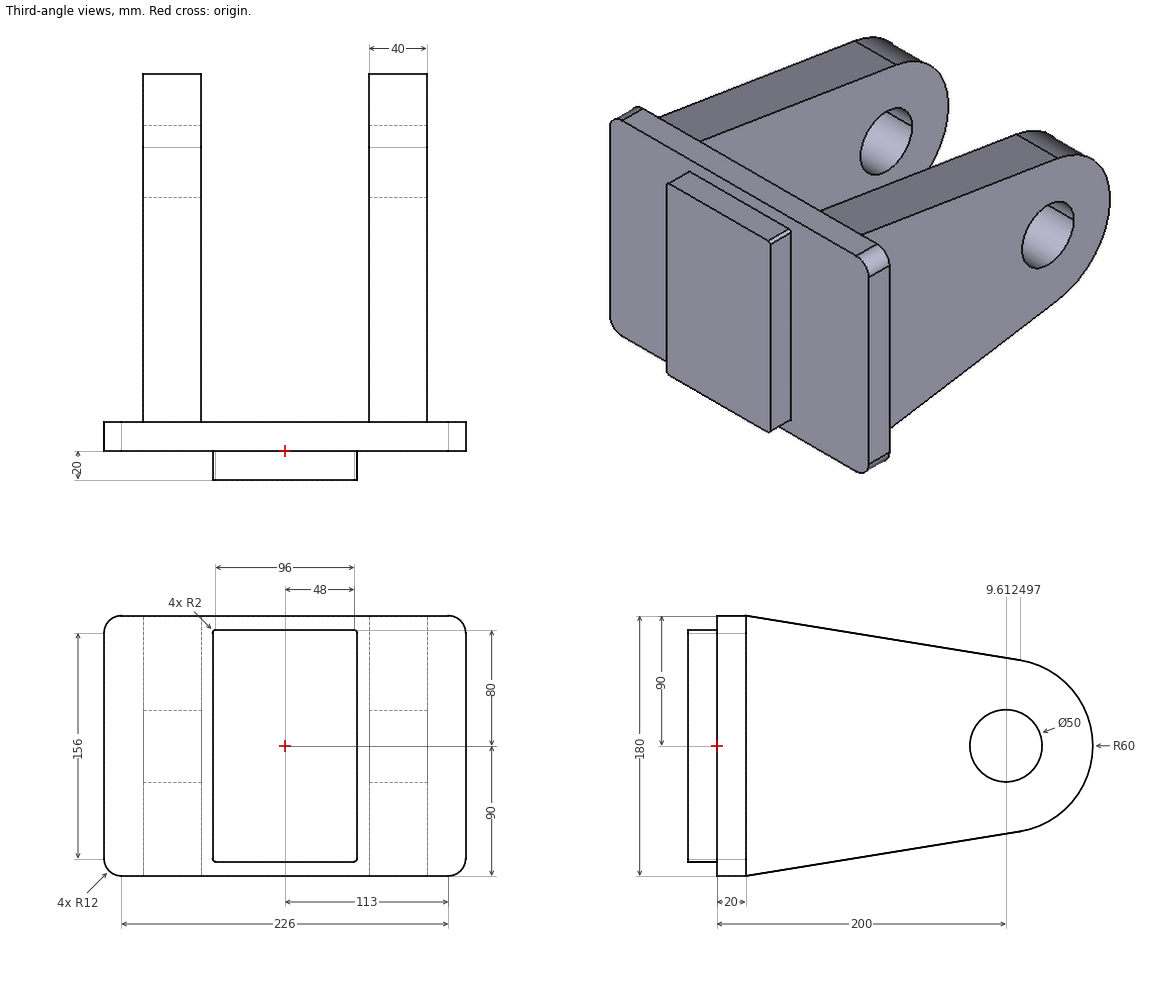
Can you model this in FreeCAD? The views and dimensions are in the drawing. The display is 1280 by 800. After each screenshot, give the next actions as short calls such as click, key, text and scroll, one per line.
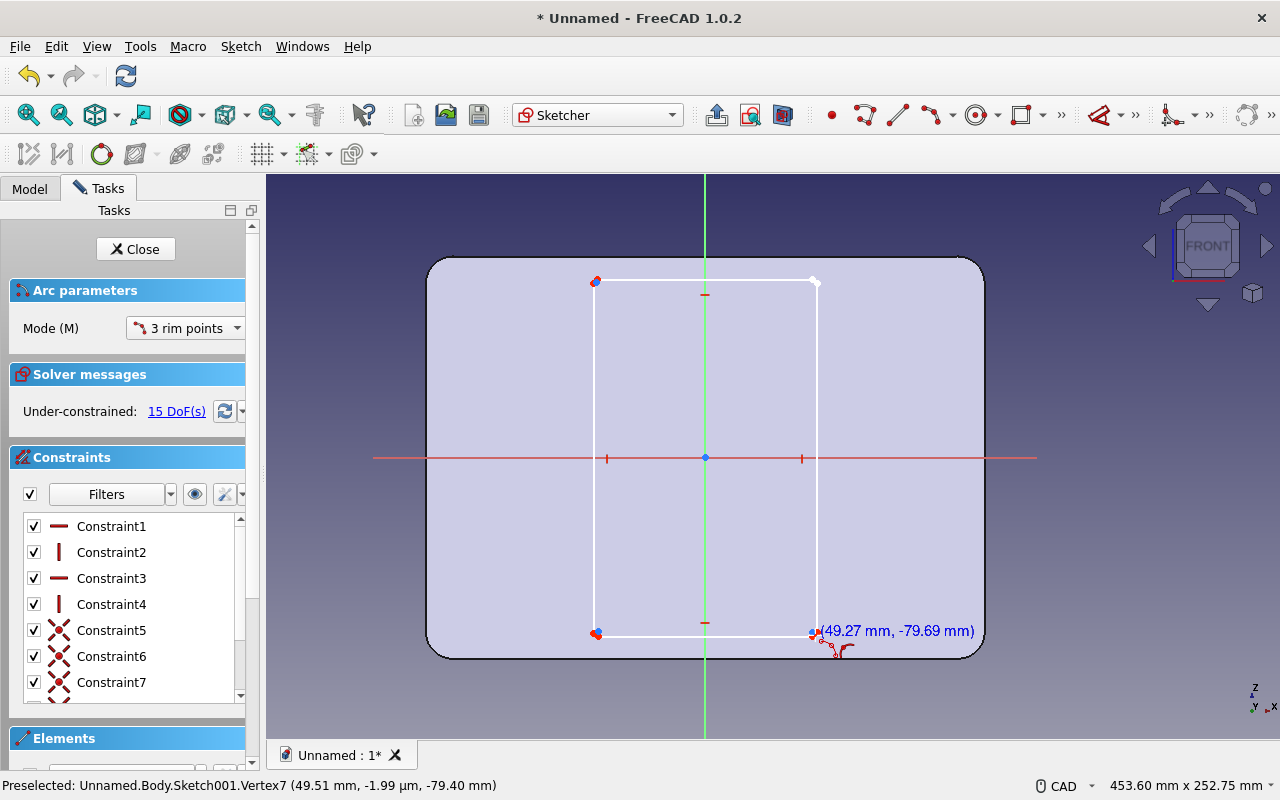
scroll(817, 283, up, 5)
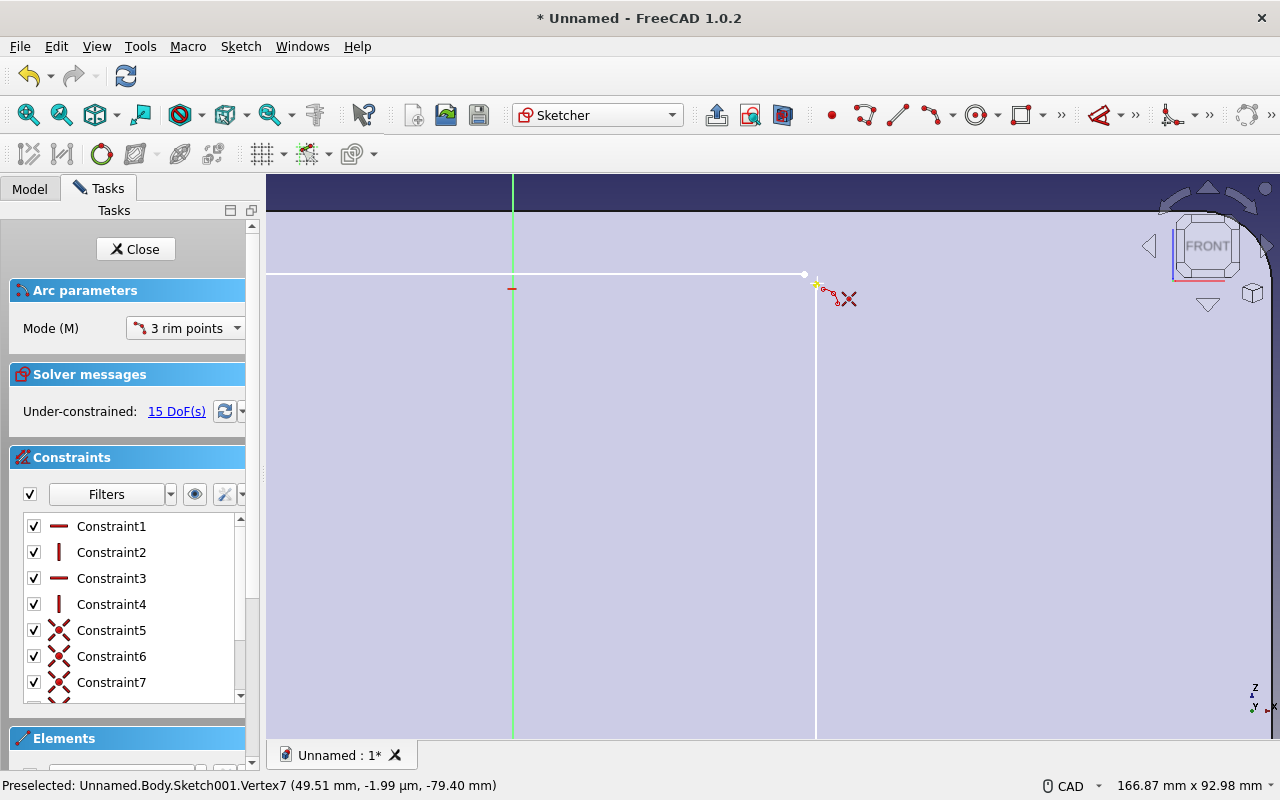
click(816, 285)
click(805, 274)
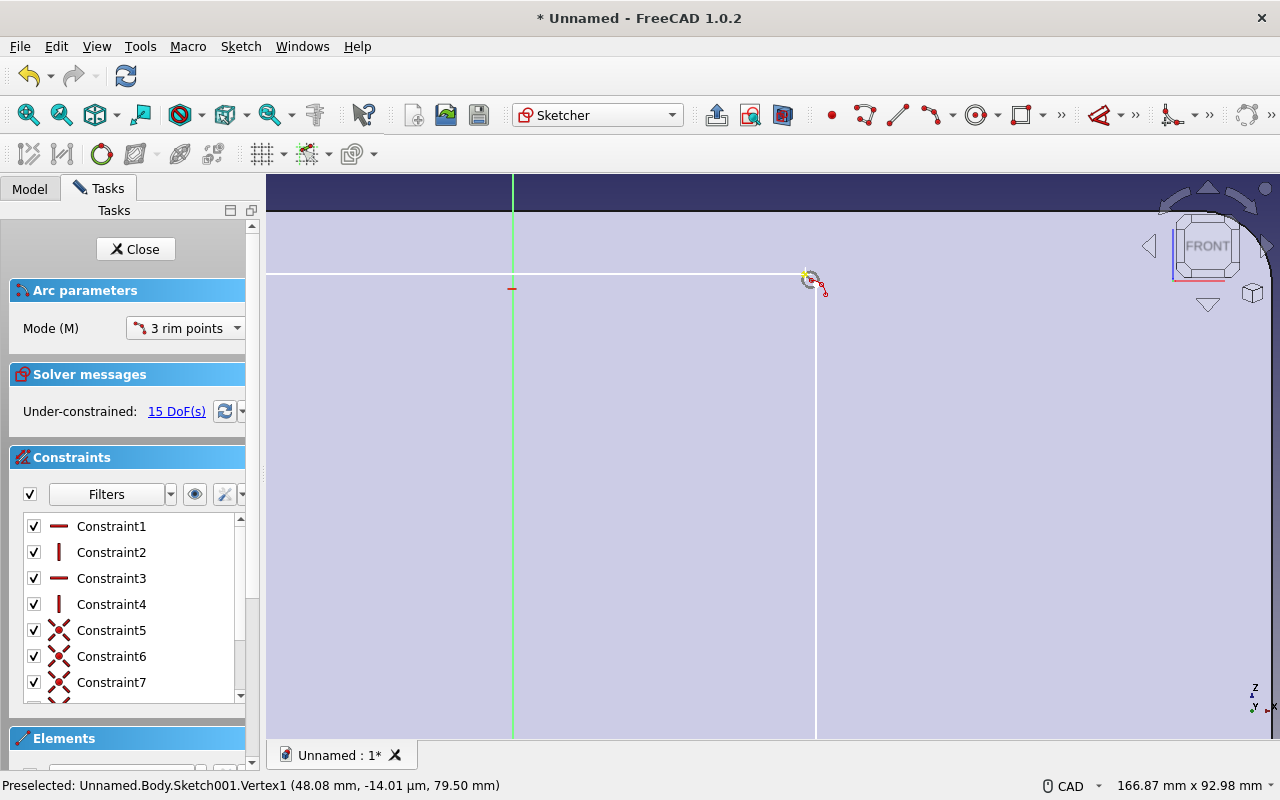
scroll(813, 275, up, 8)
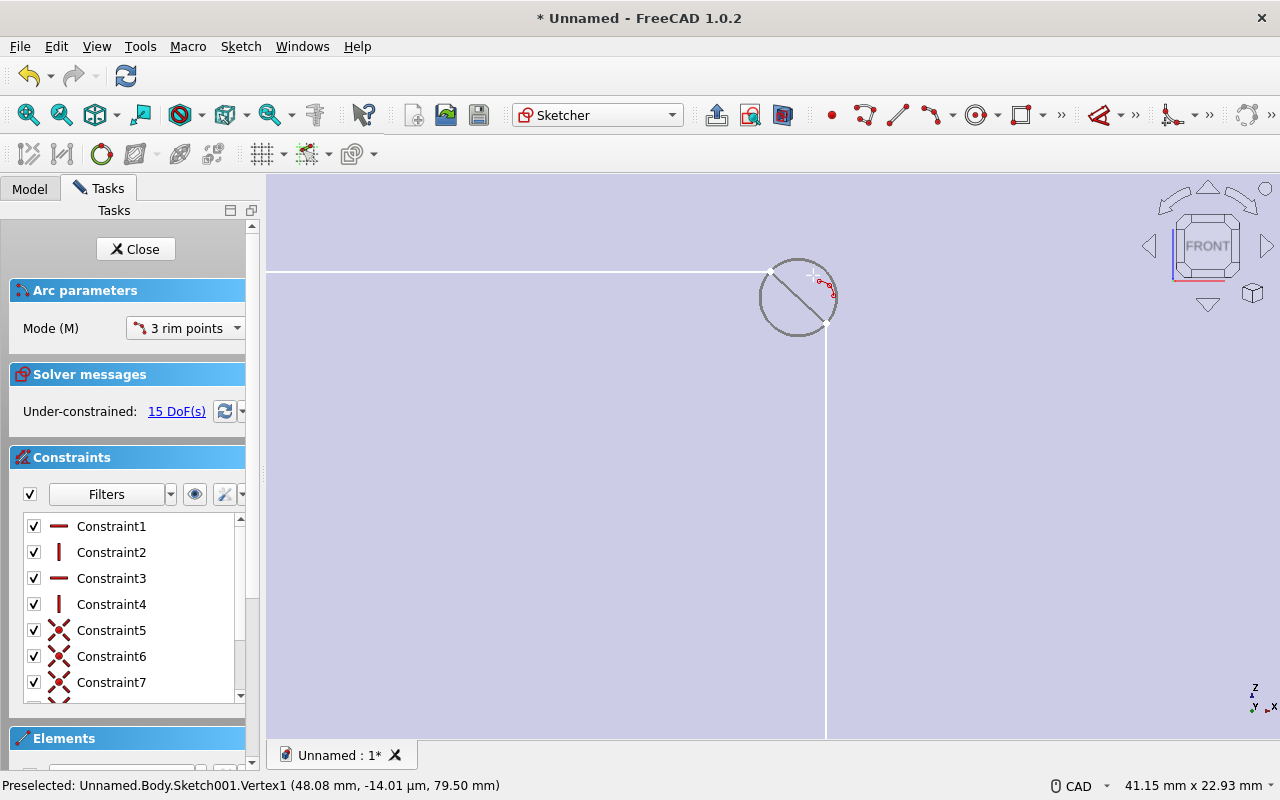
click(810, 274)
key(Escape)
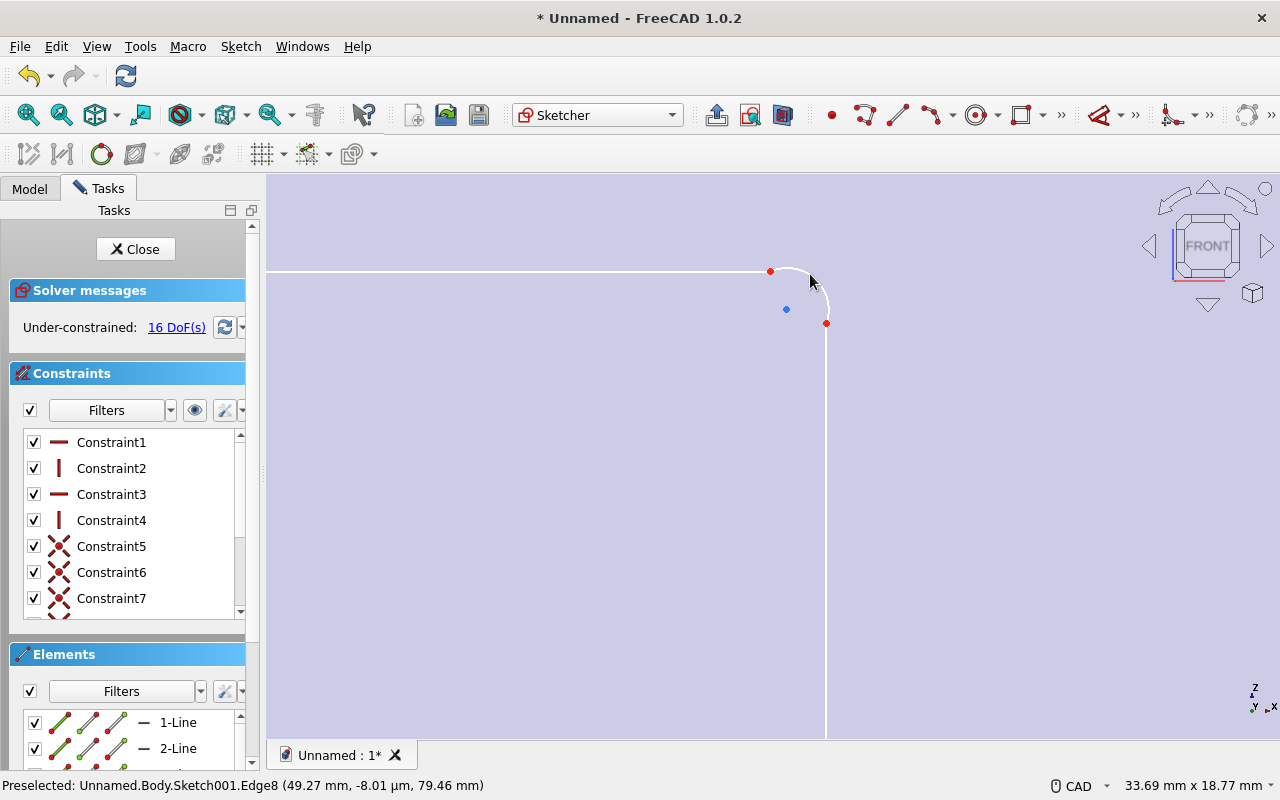
scroll(815, 279, down, 13)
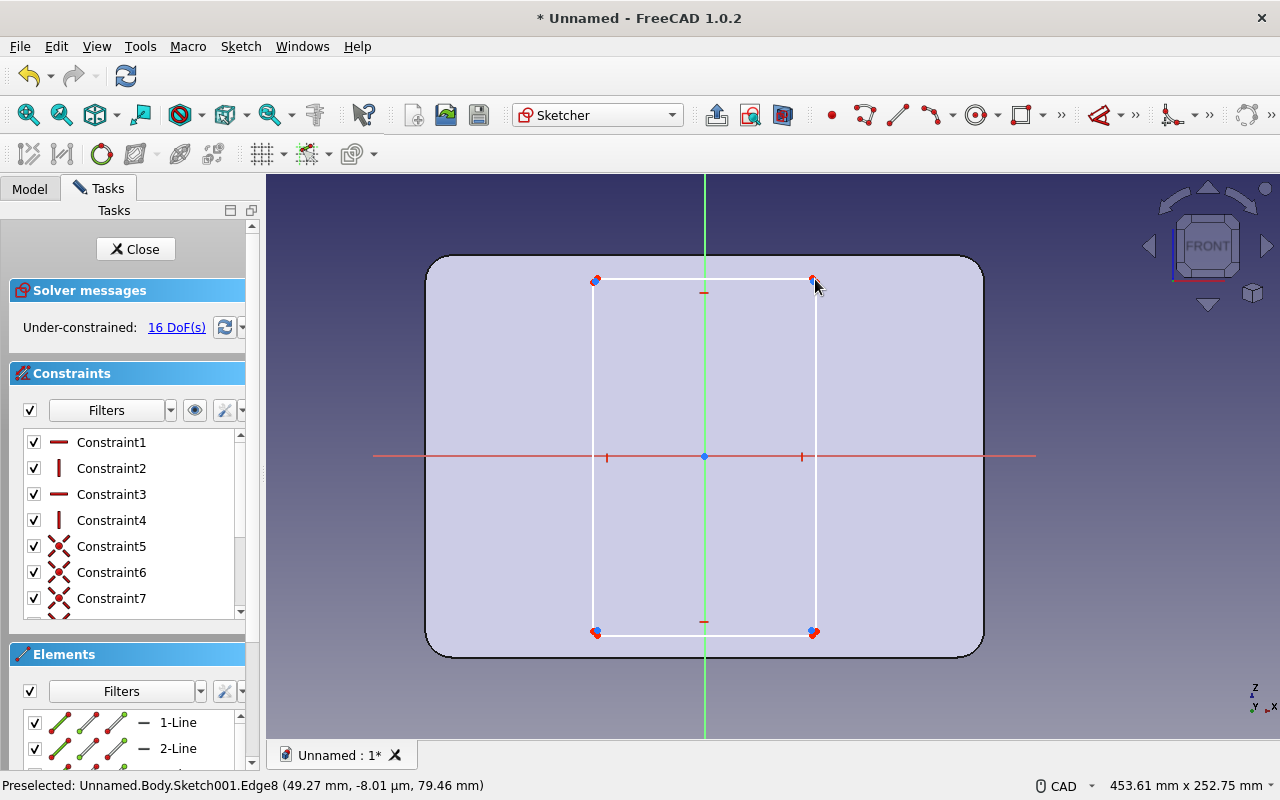
click(748, 279)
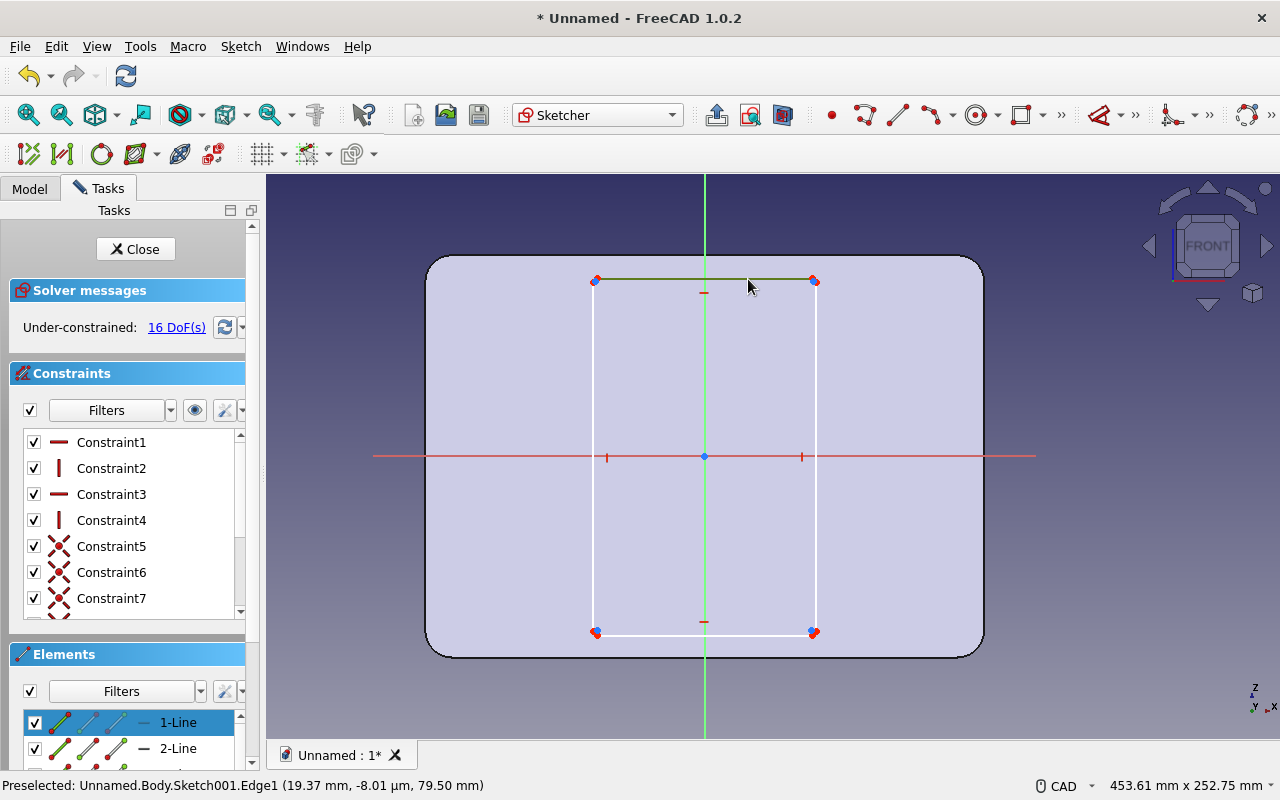
scroll(594, 279, up, 8)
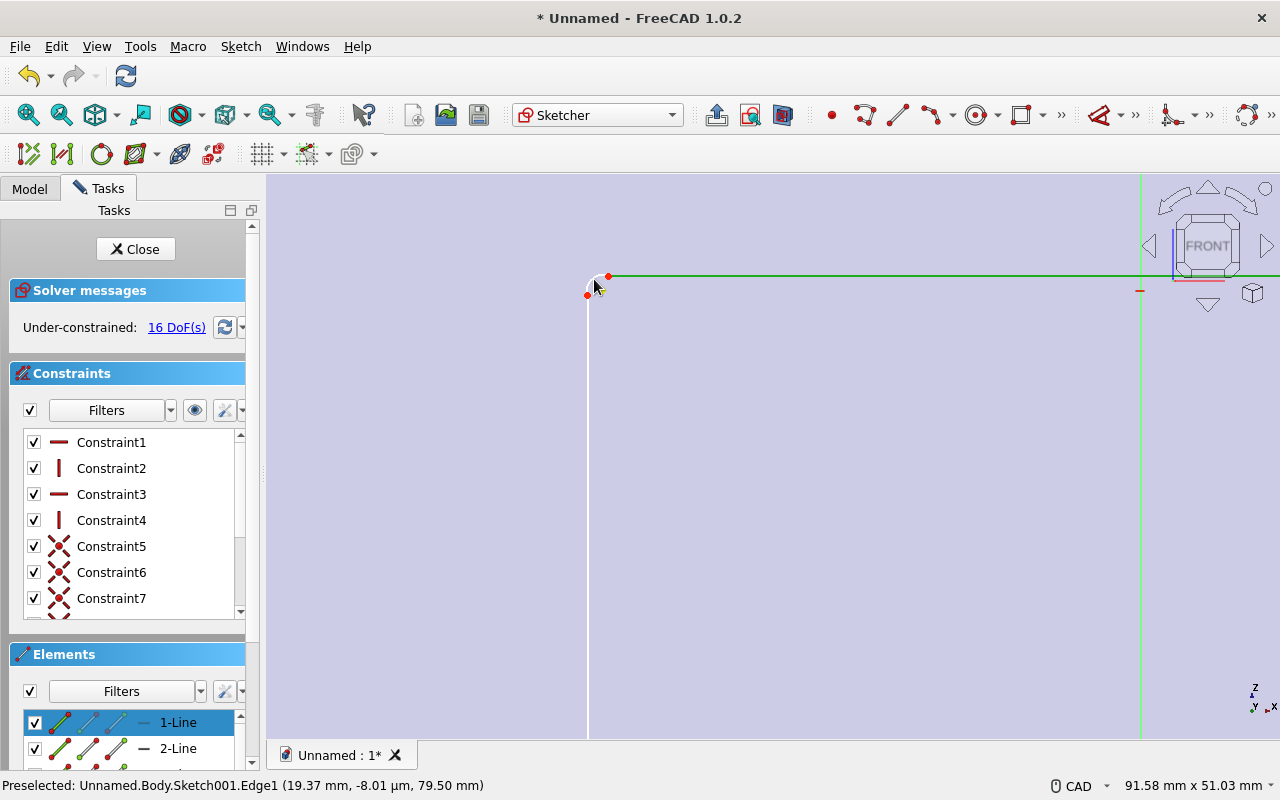
click(592, 279)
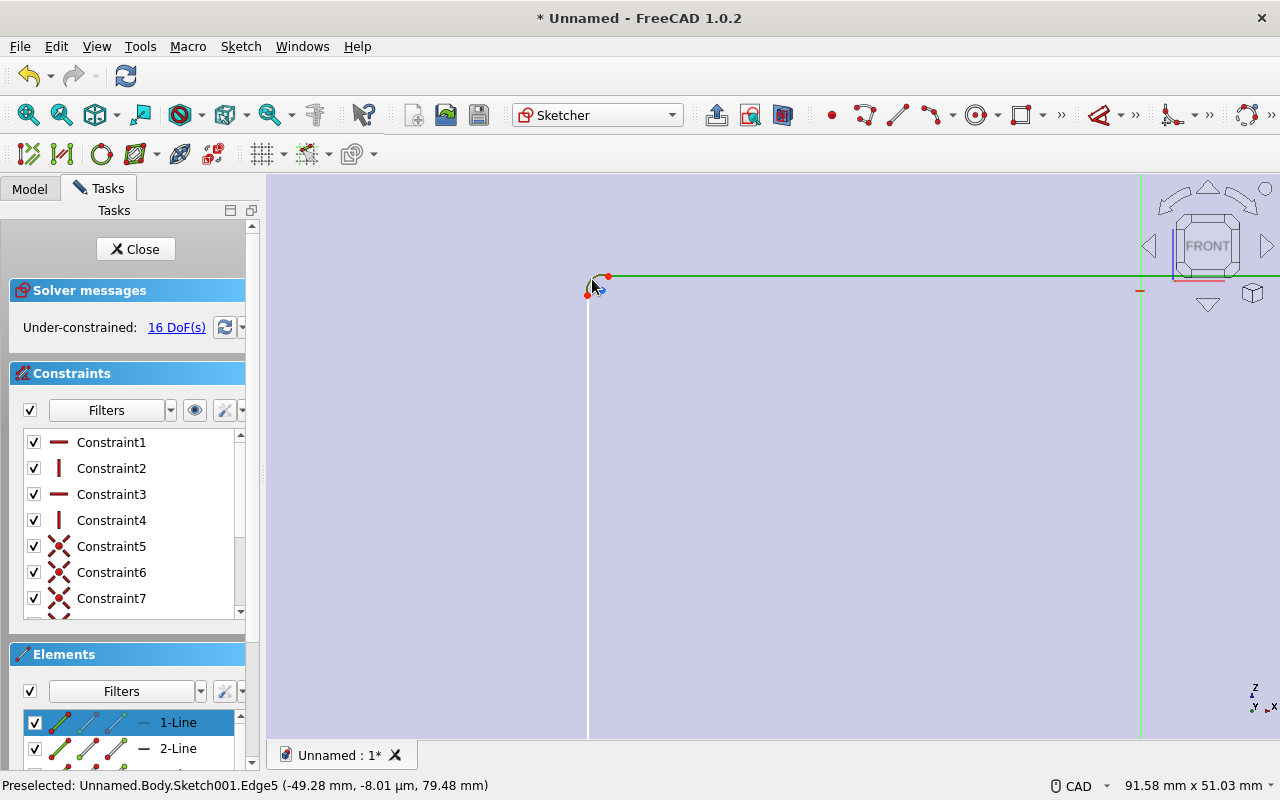
key(t)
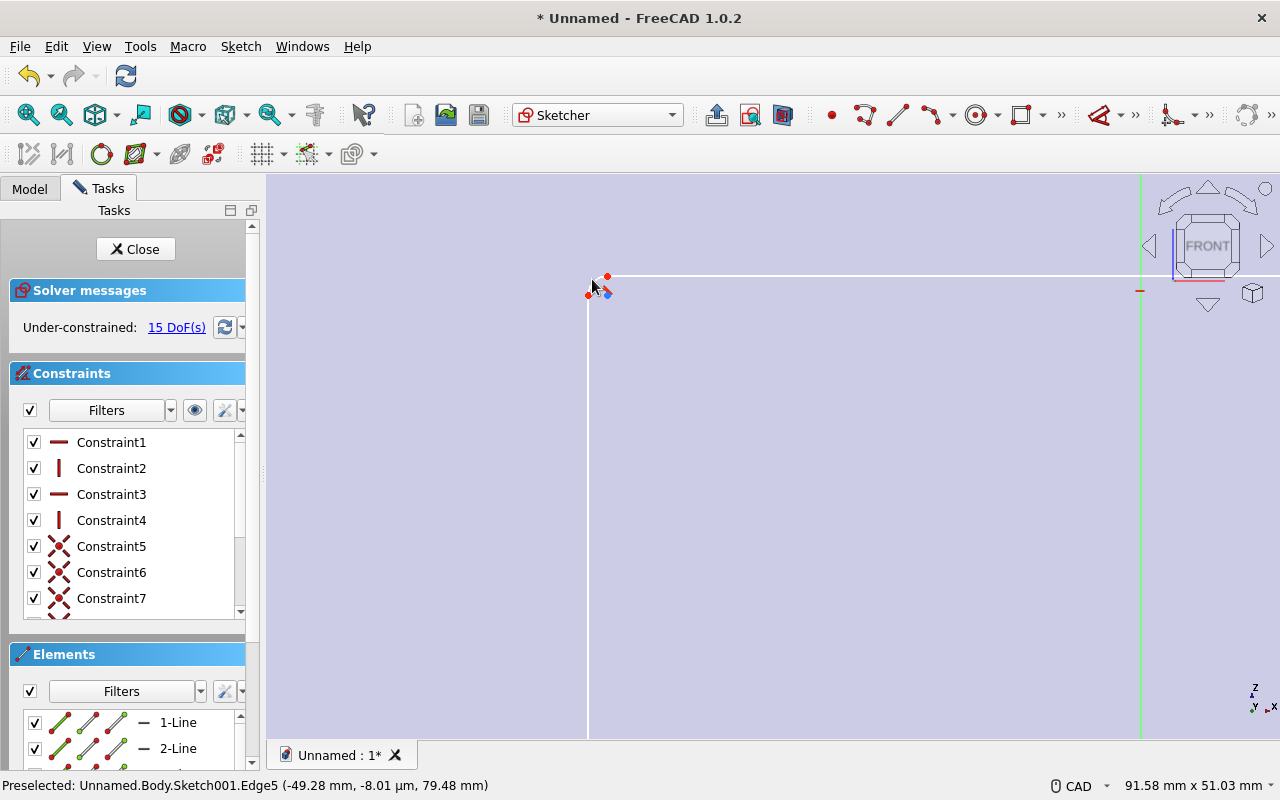
scroll(594, 279, down, 8)